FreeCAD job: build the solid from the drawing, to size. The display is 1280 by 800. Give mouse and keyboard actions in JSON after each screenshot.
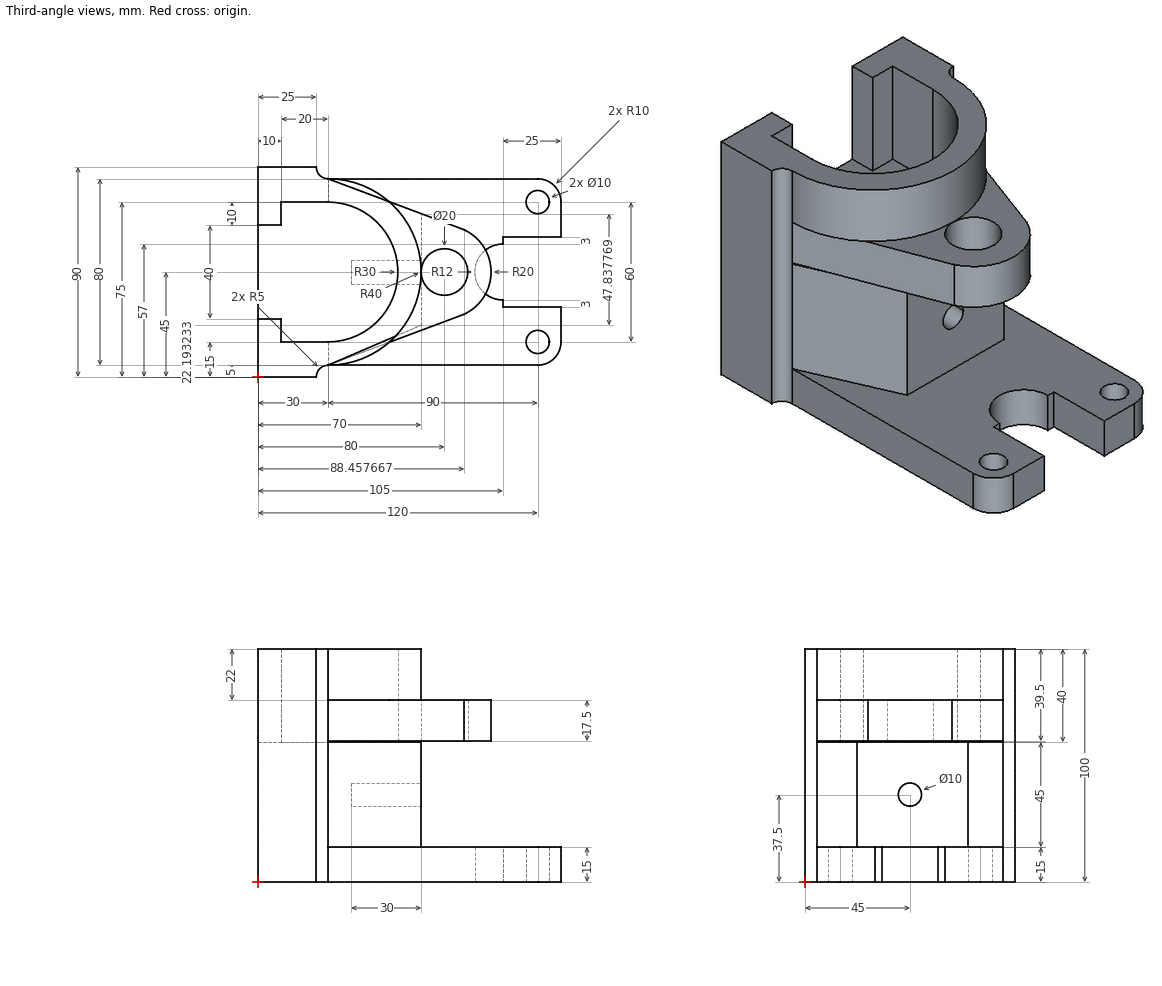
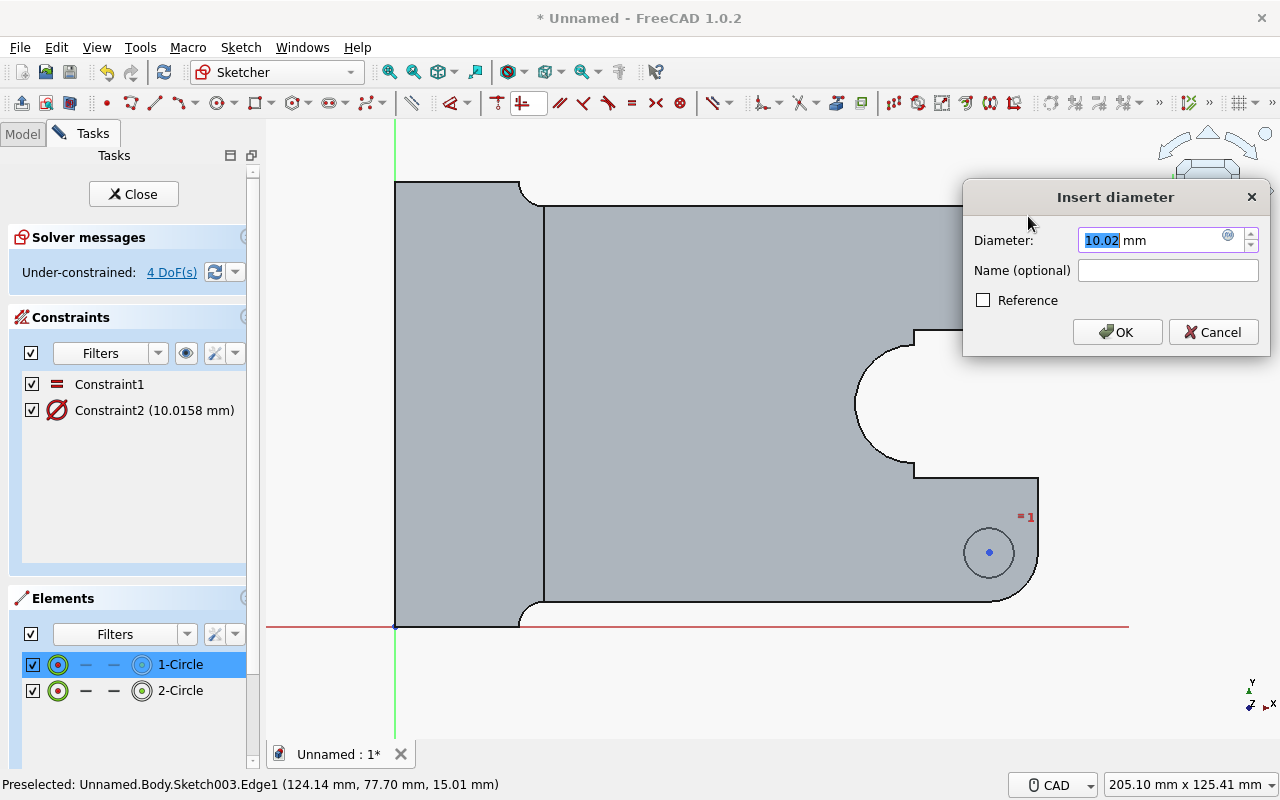
{"action": "type", "text": "10"}
{"action": "key", "text": "Return"}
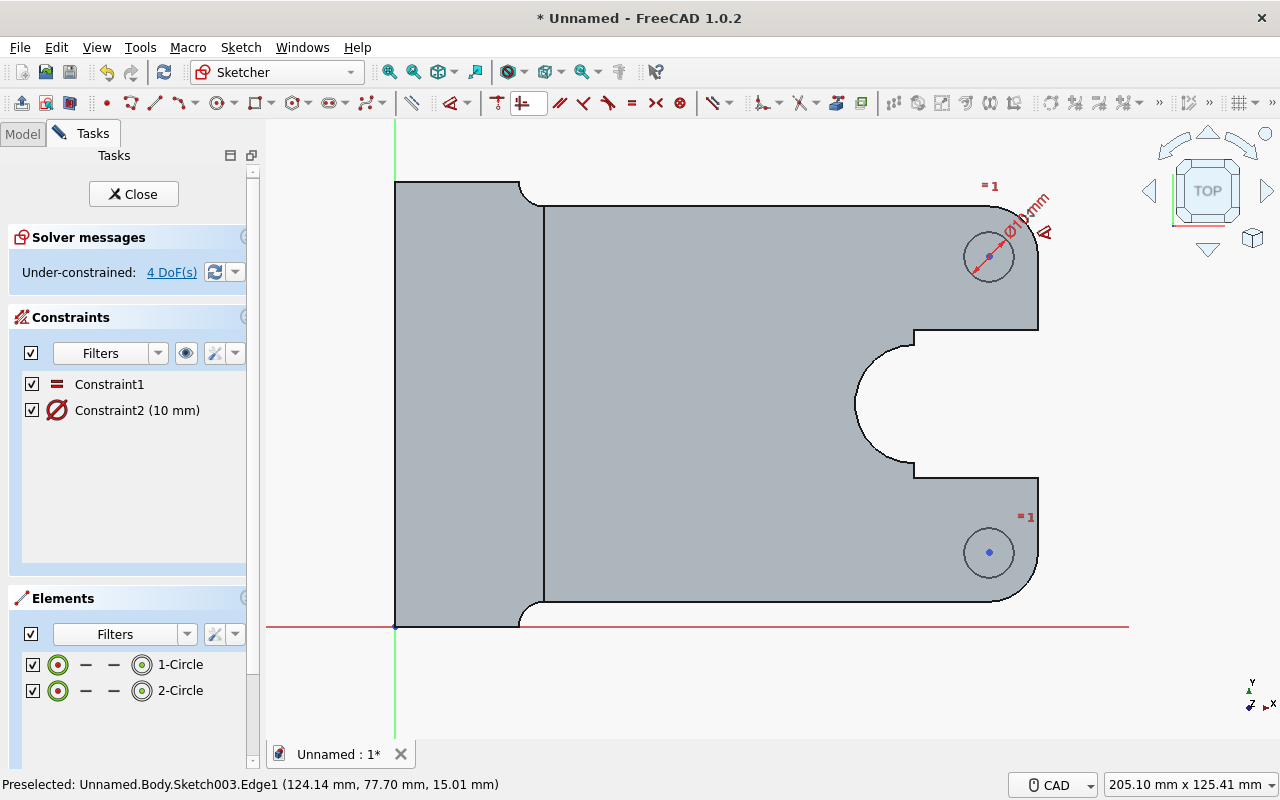
{"action": "left_click", "coordinate": [989, 257]}
{"action": "left_click", "coordinate": [361, 442]}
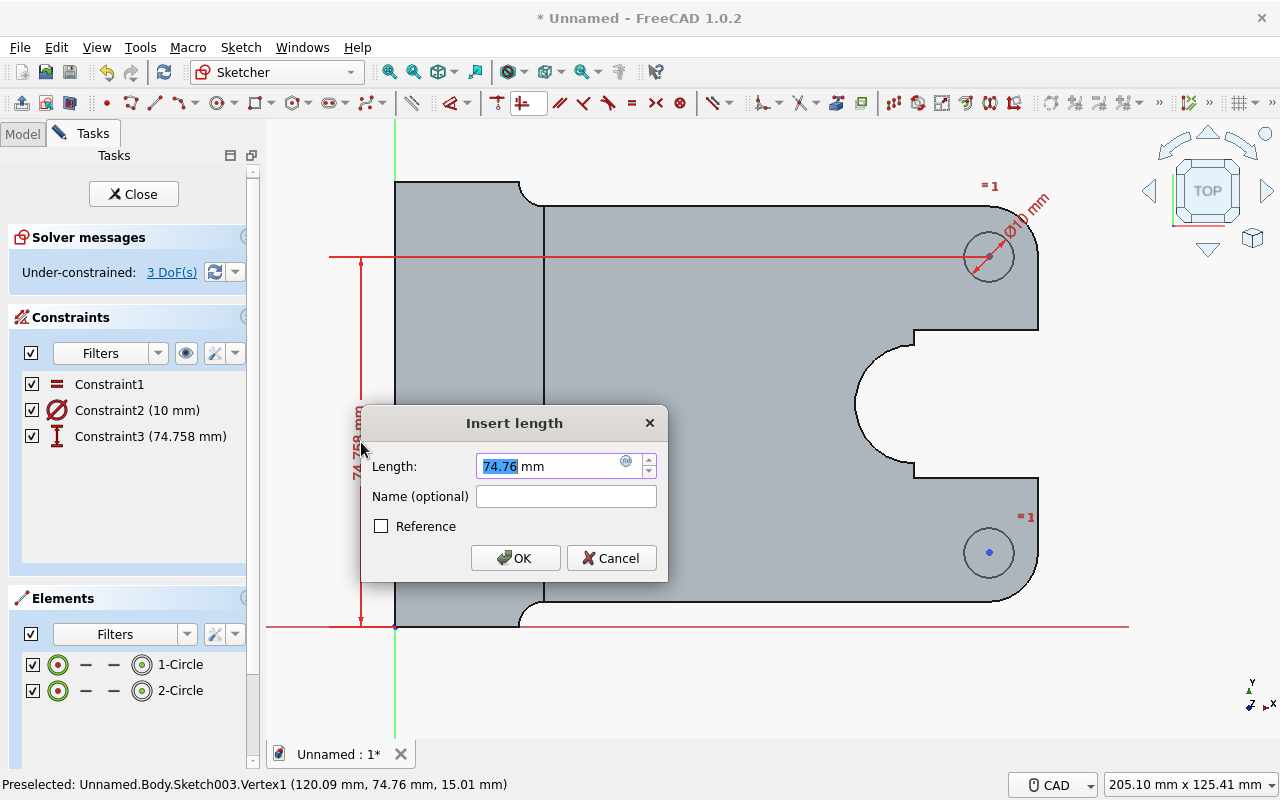
{"action": "type", "text": "75"}
{"action": "key", "text": "Return"}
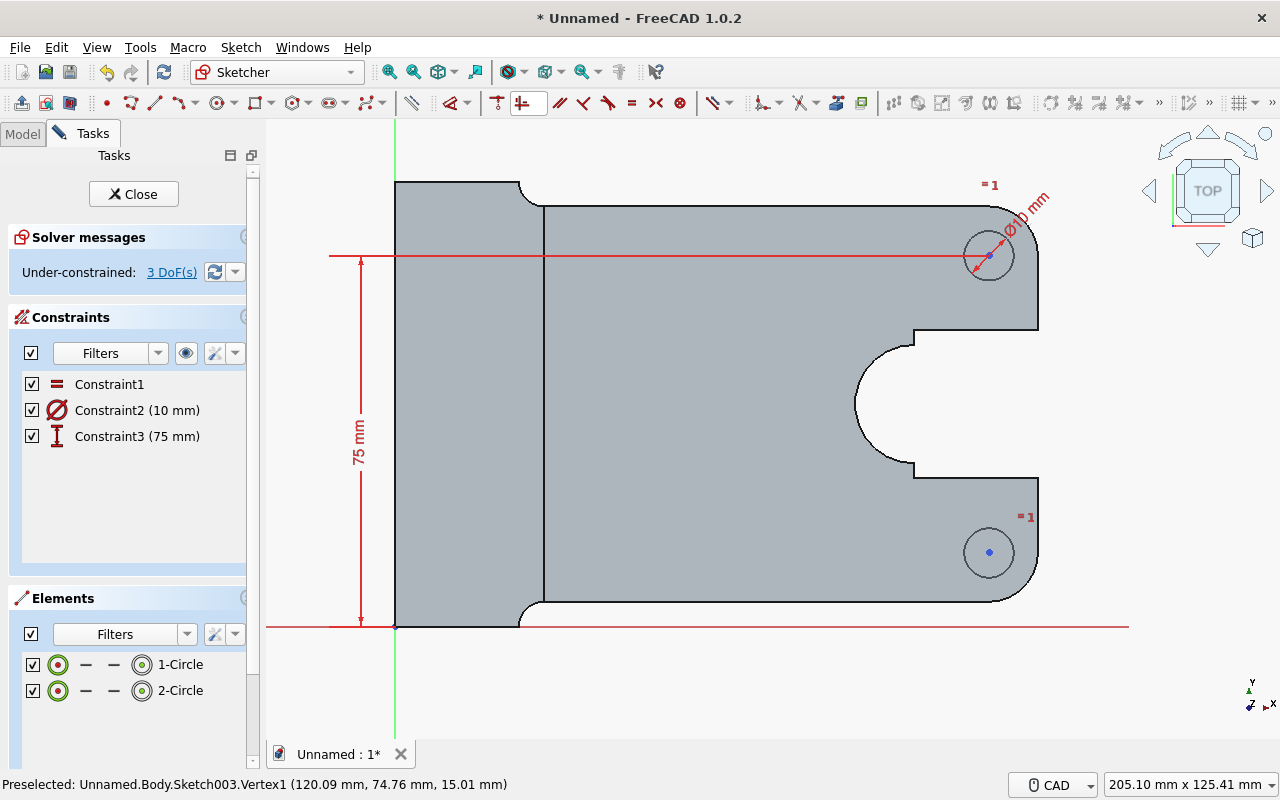
{"action": "left_click", "coordinate": [989, 553]}
{"action": "left_click", "coordinate": [361, 590]}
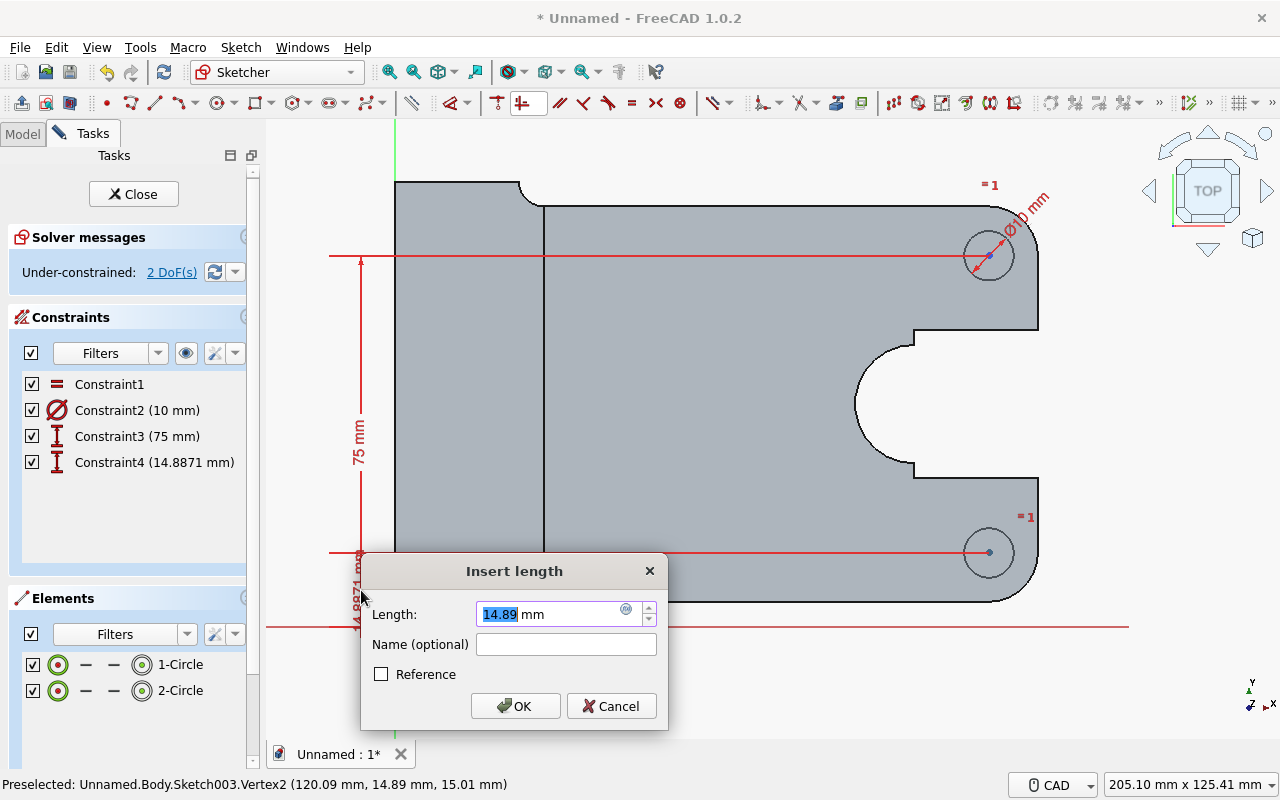
{"action": "type", "text": "15"}
{"action": "key", "text": "Return"}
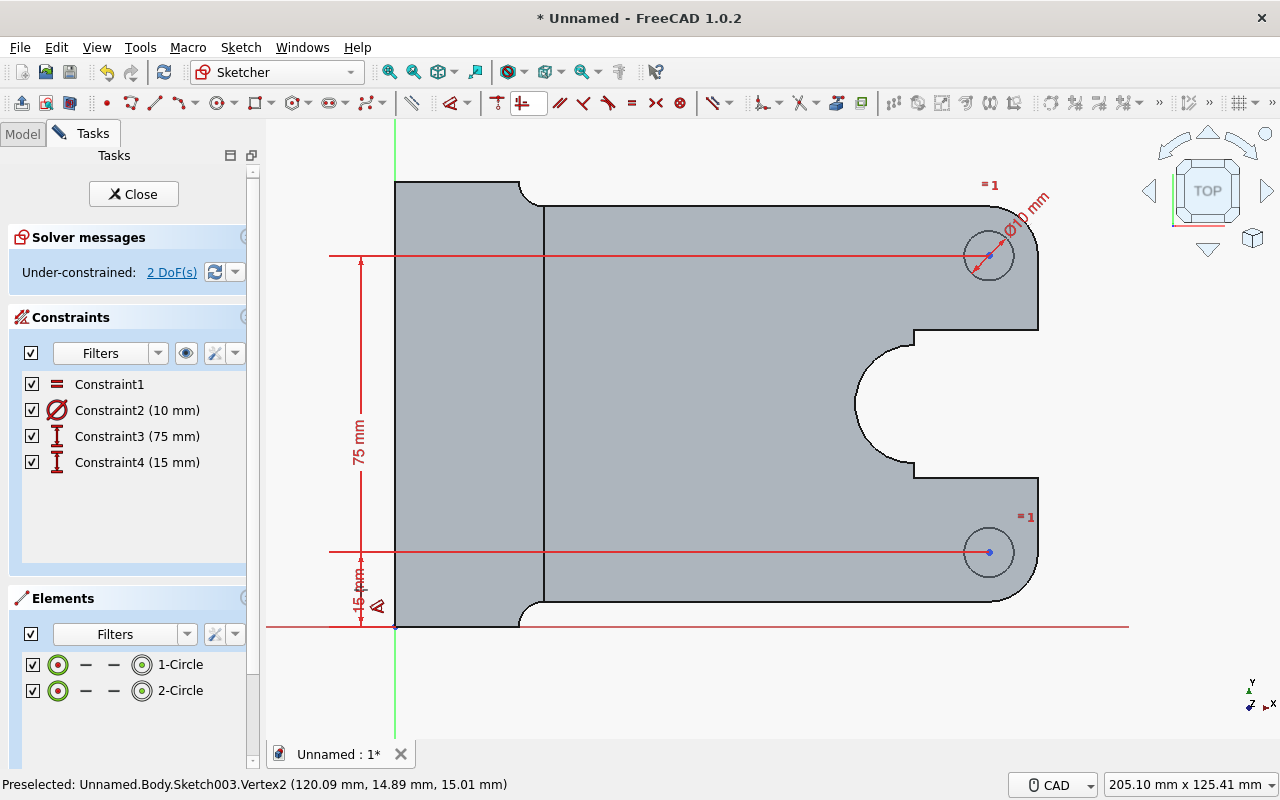
{"action": "left_click", "coordinate": [989, 256]}
{"action": "left_click", "coordinate": [692, 661]}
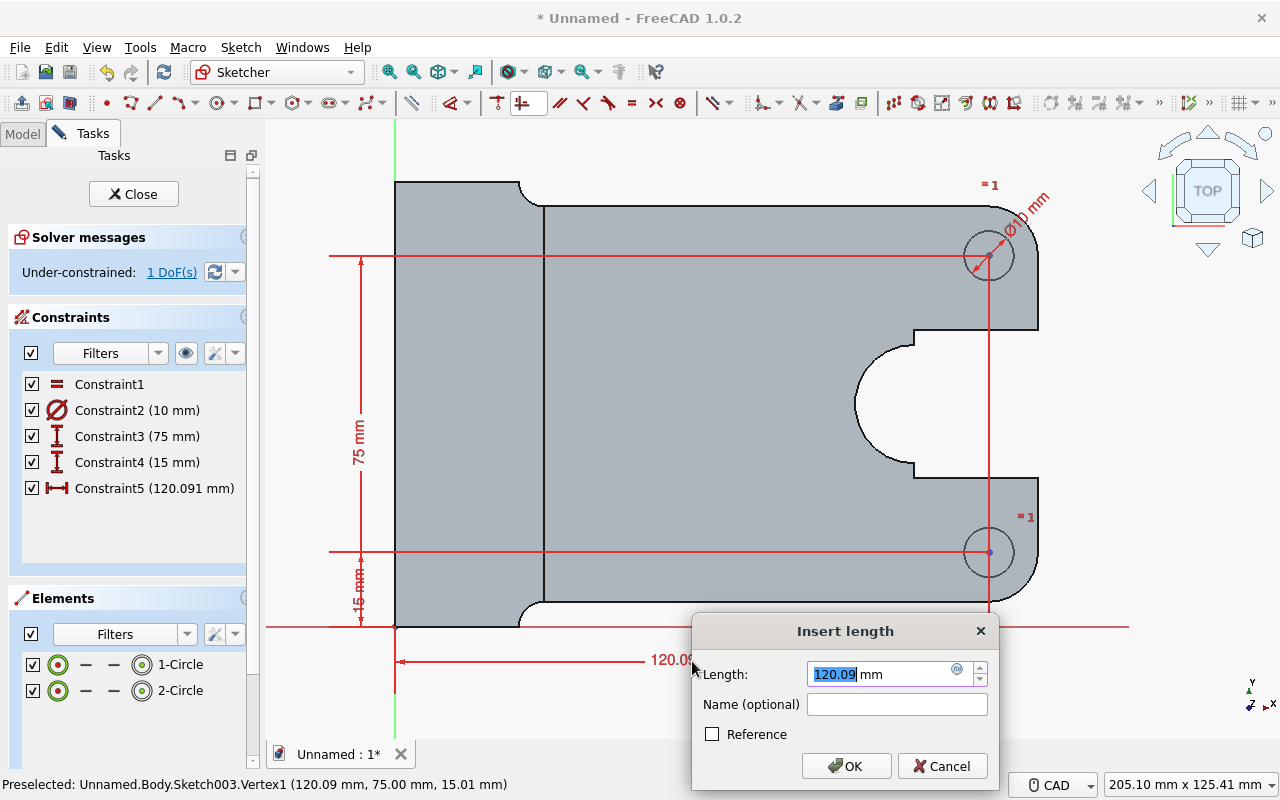
{"action": "type", "text": "120"}
{"action": "key", "text": "Return"}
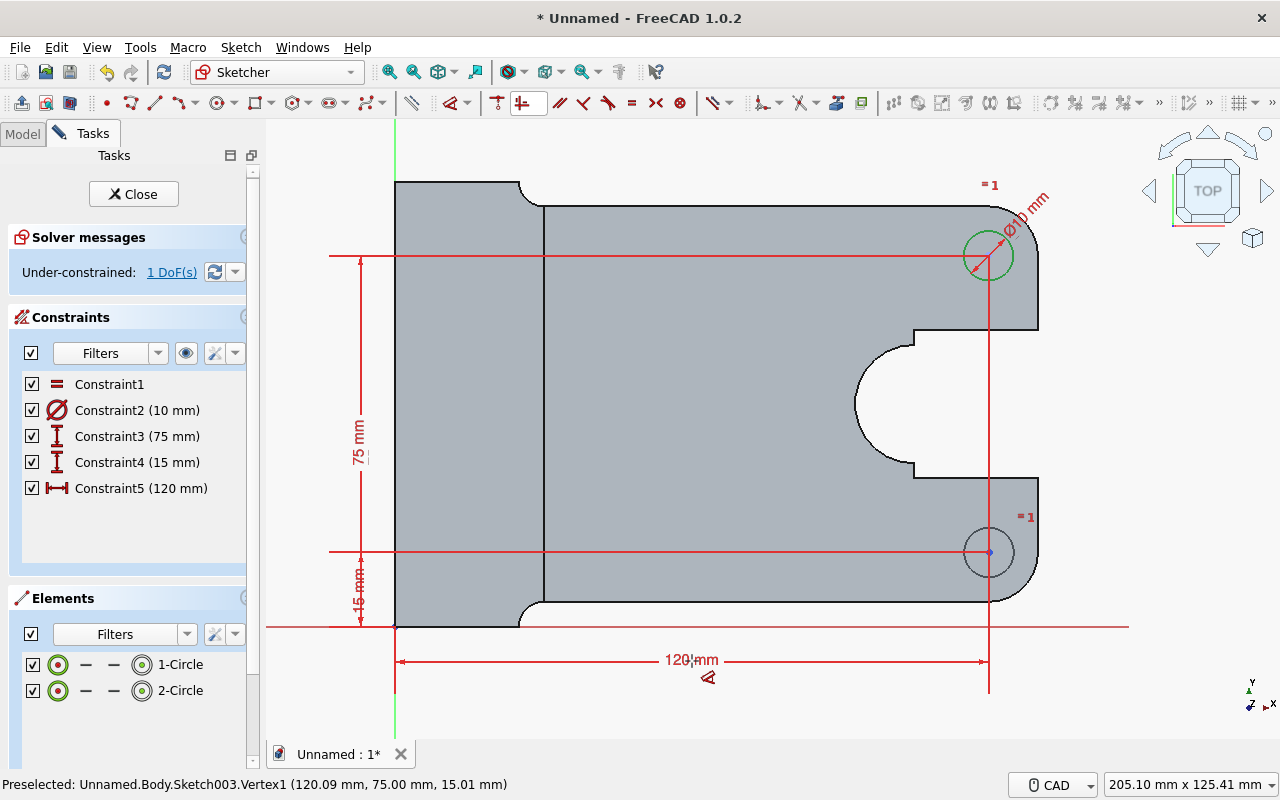
{"action": "left_click", "coordinate": [989, 552]}
{"action": "left_click", "coordinate": [556, 661]}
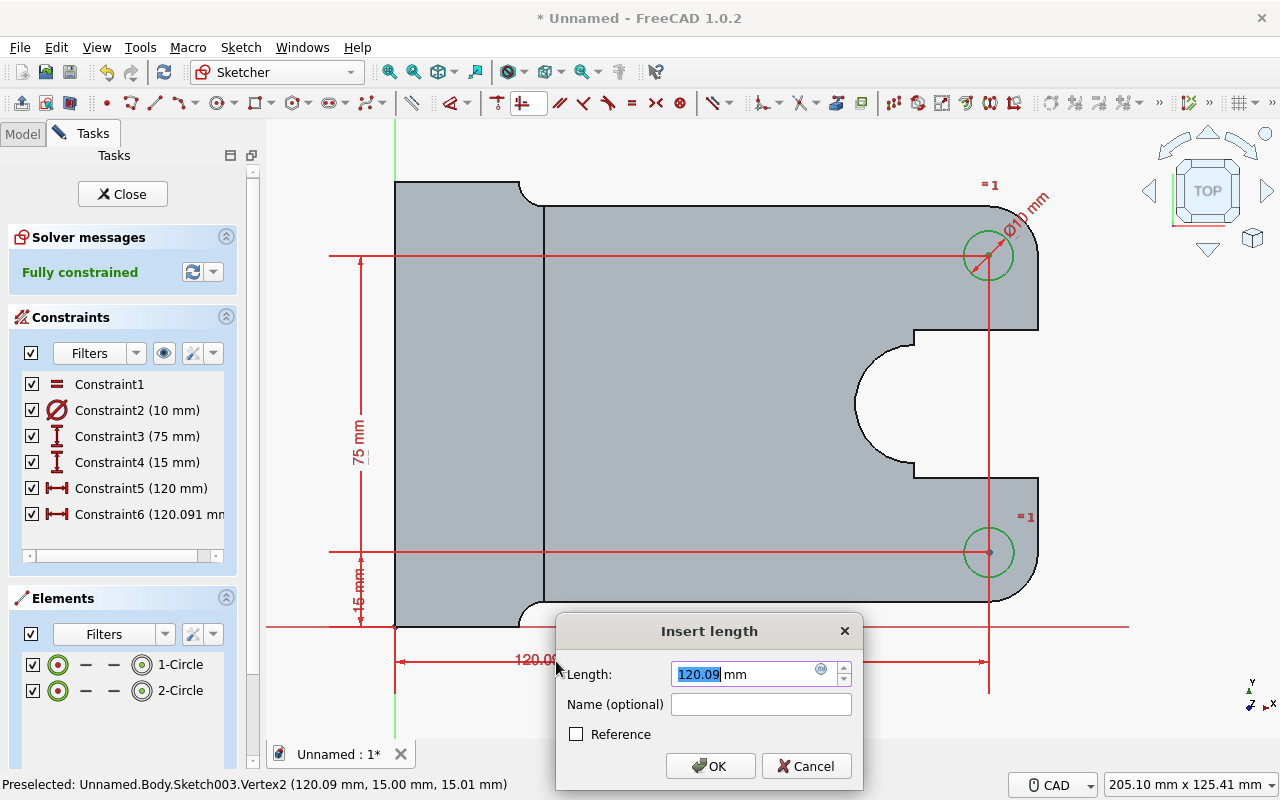
{"action": "type", "text": "120"}
{"action": "key", "text": "Return"}
{"action": "key", "text": "Escape"}